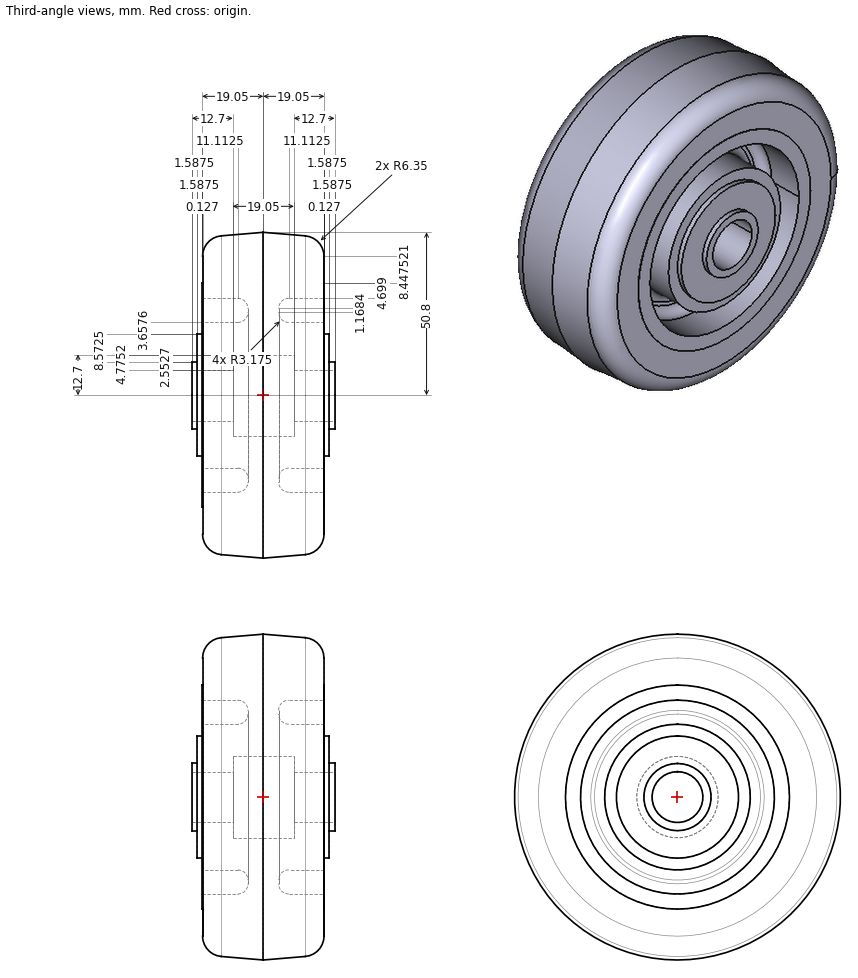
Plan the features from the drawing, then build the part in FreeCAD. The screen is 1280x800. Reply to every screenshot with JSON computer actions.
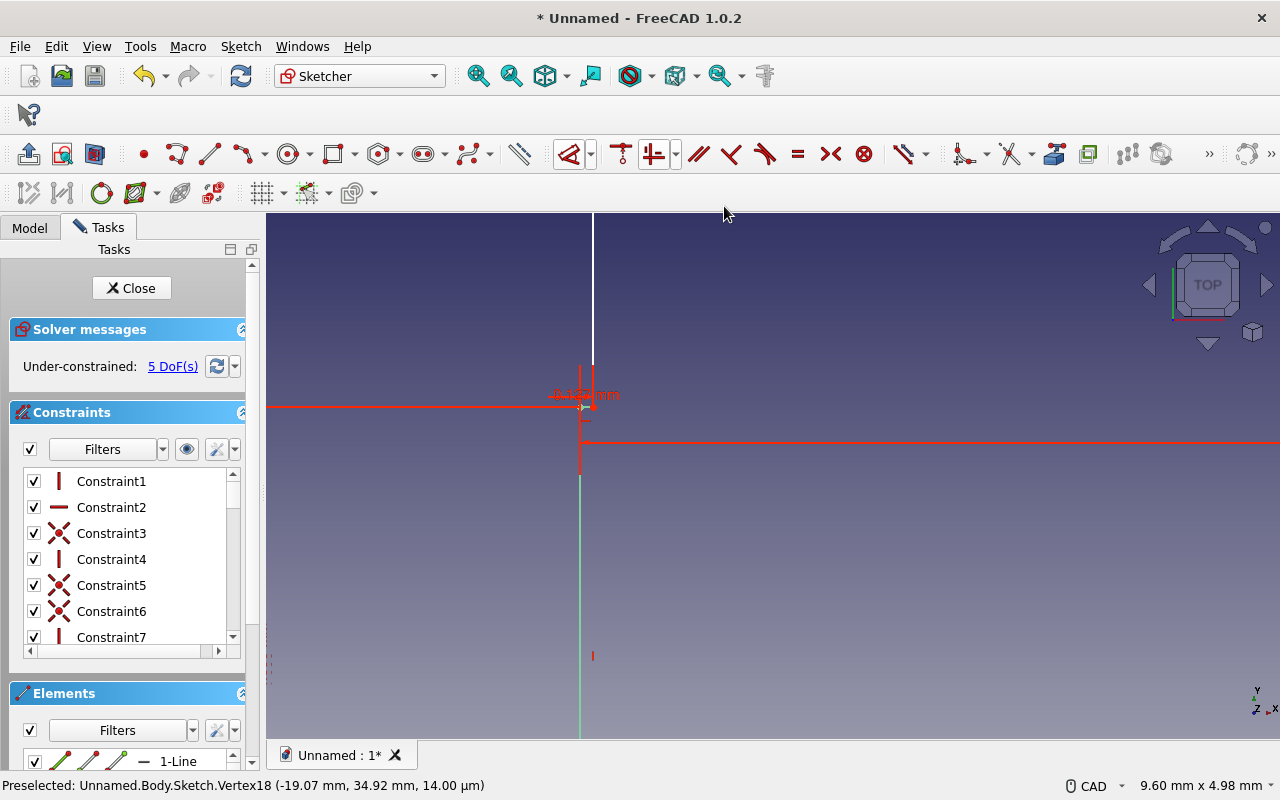
{"action": "scroll", "coordinate": [582, 415], "scroll_direction": "down", "scroll_amount": 14}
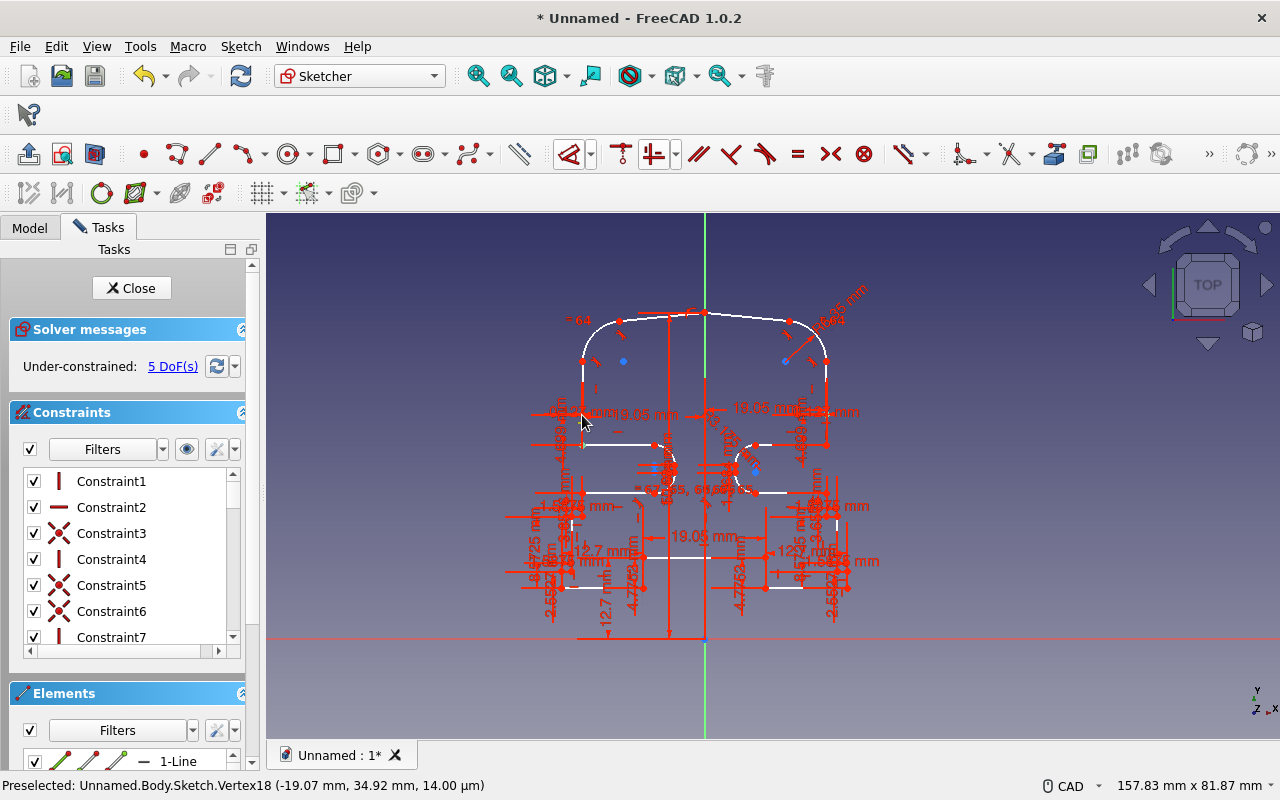
{"action": "left_click", "coordinate": [582, 493]}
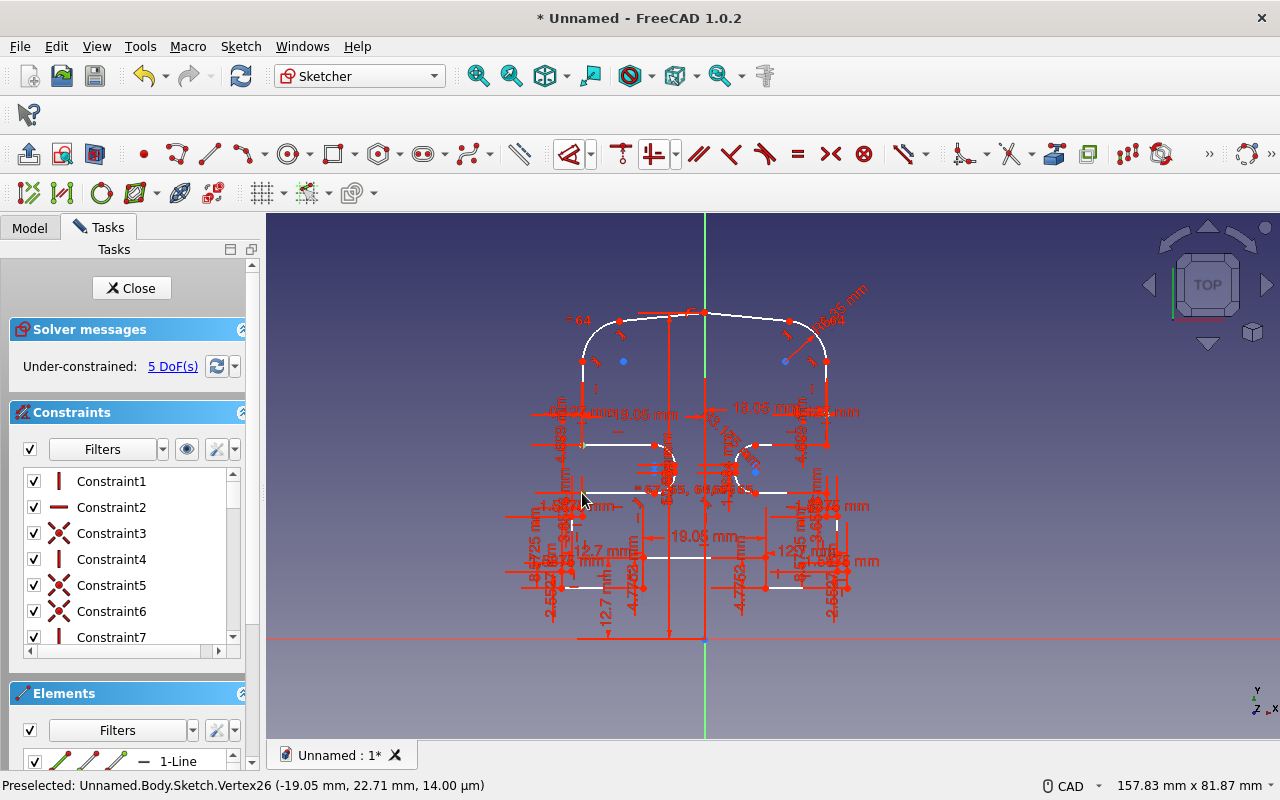
{"action": "left_click", "coordinate": [590, 154]}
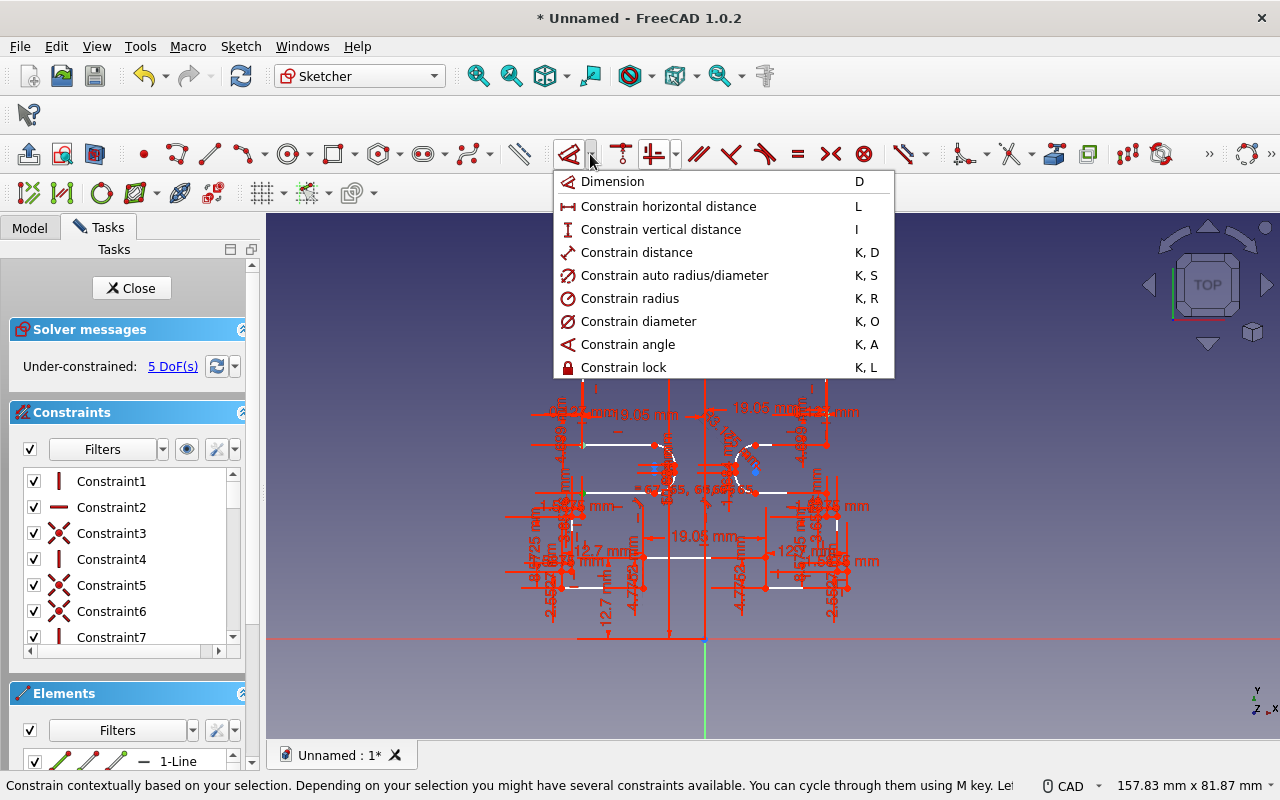
{"action": "left_click", "coordinate": [724, 206]}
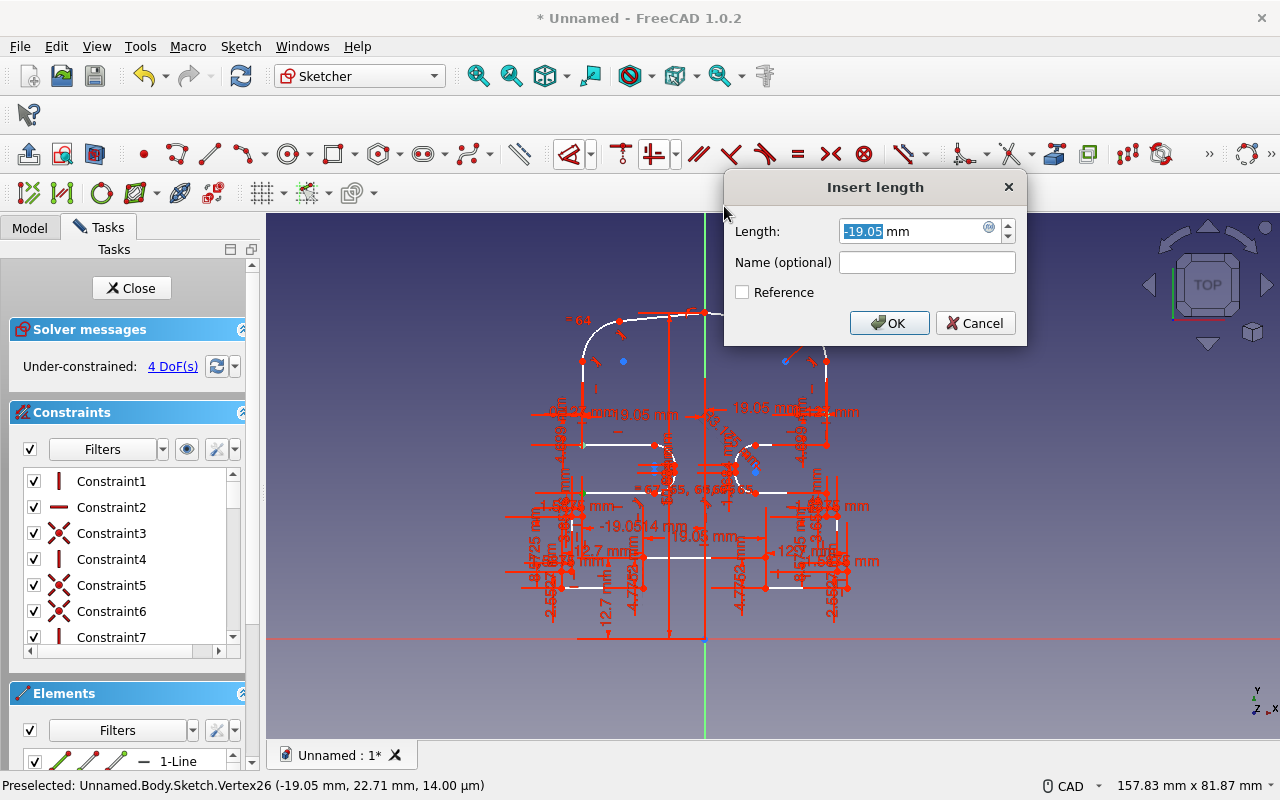
{"action": "type", "text": "-19.05"}
{"action": "key", "text": "Return"}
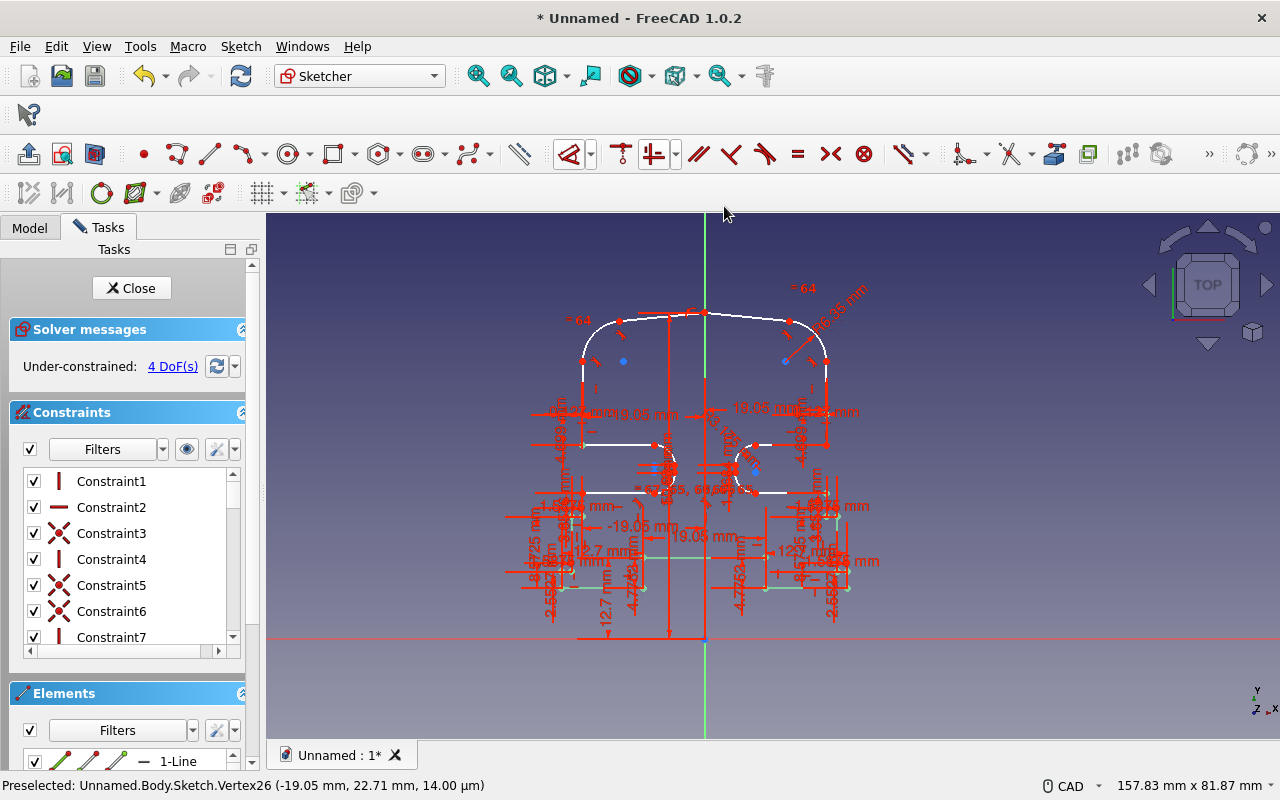
{"action": "left_click", "coordinate": [777, 445]}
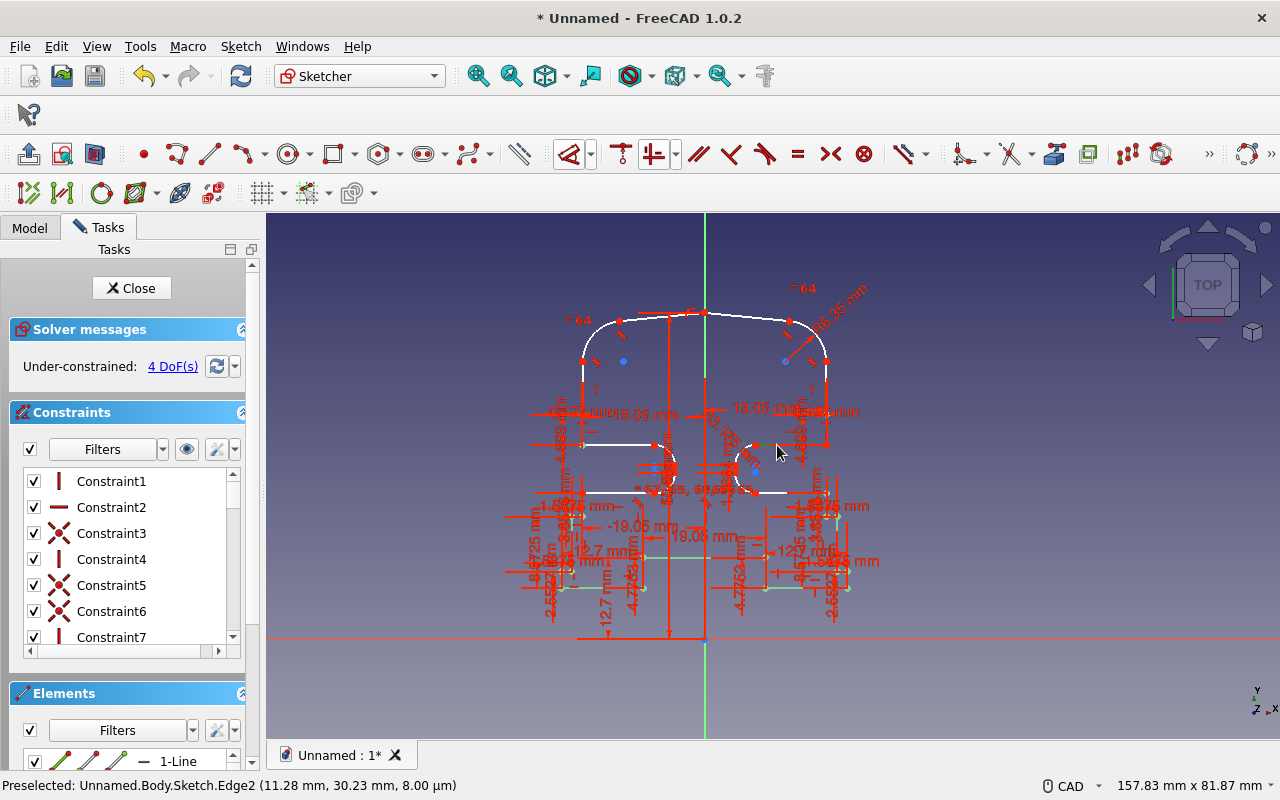
{"action": "left_click", "coordinate": [590, 154]}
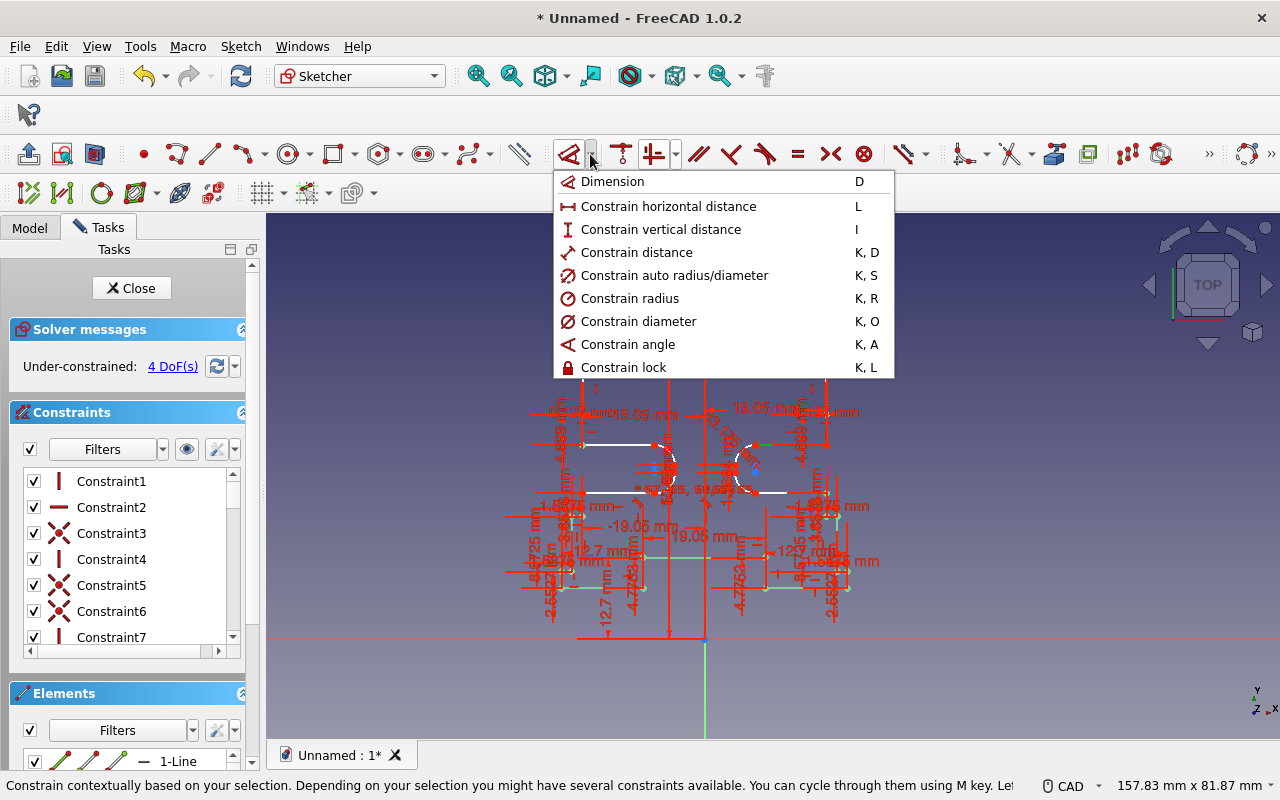
{"action": "left_click", "coordinate": [724, 206]}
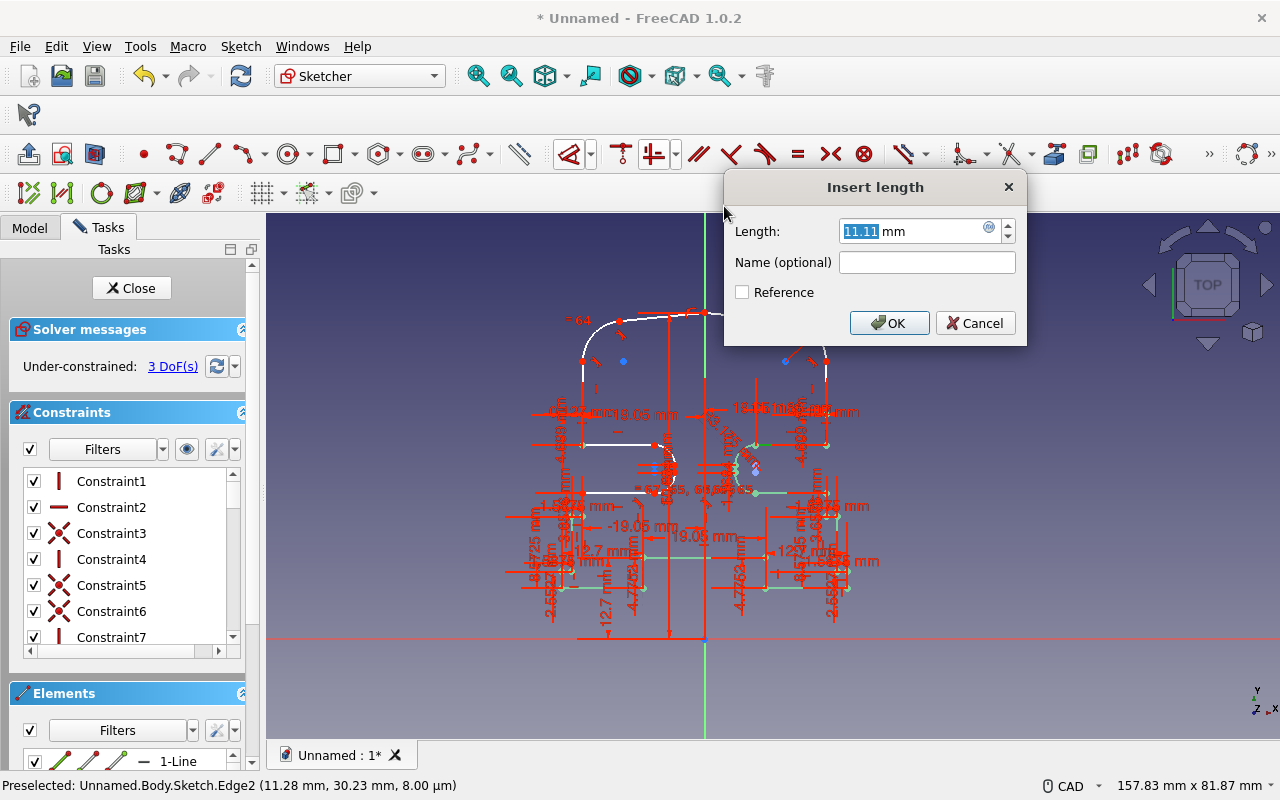
{"action": "type", "text": "11.1125"}
{"action": "key", "text": "Return"}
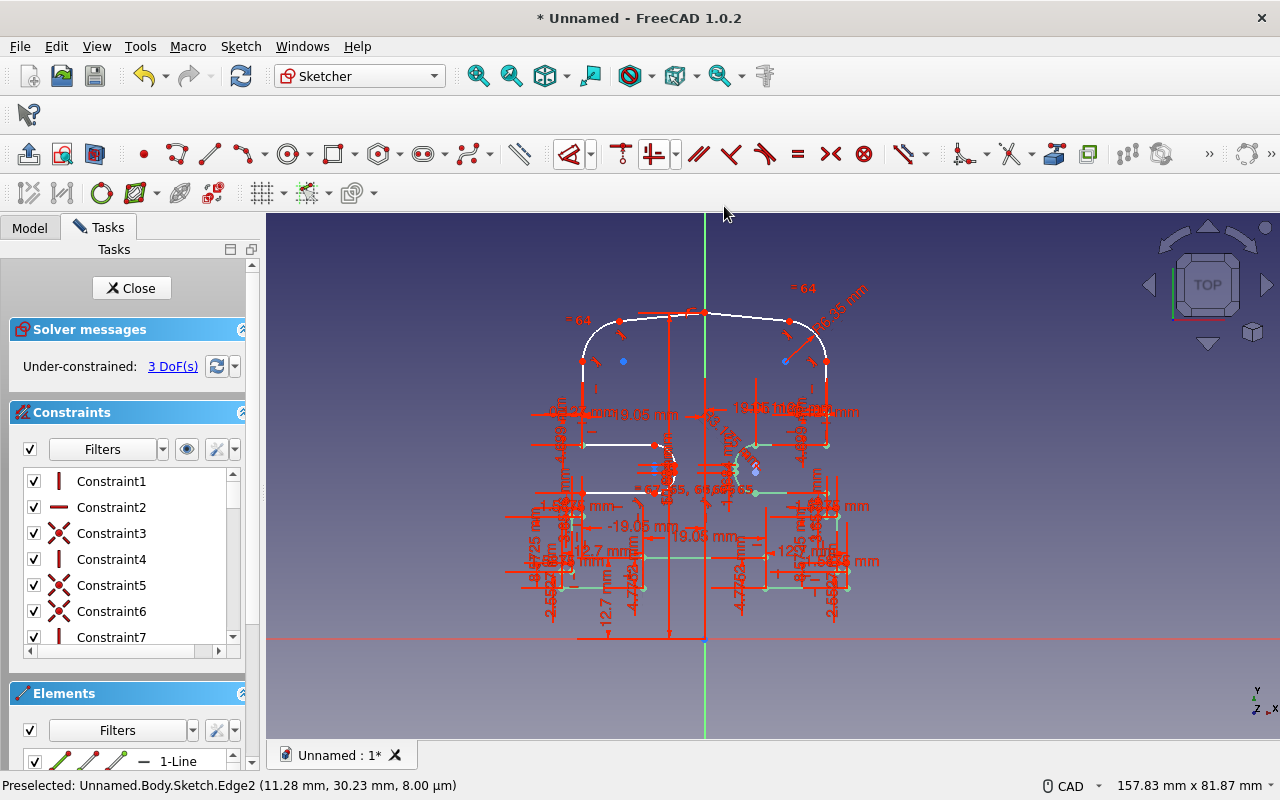
{"action": "left_click", "coordinate": [604, 445]}